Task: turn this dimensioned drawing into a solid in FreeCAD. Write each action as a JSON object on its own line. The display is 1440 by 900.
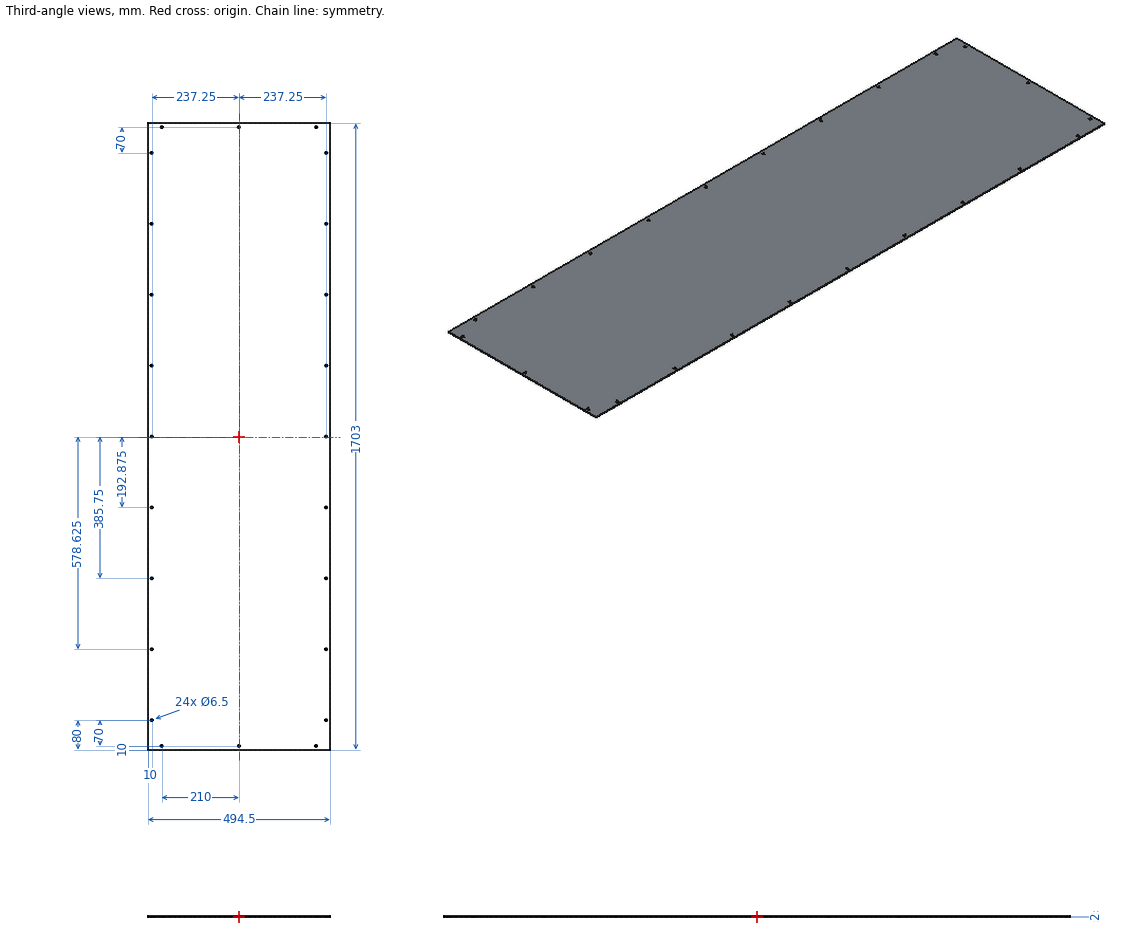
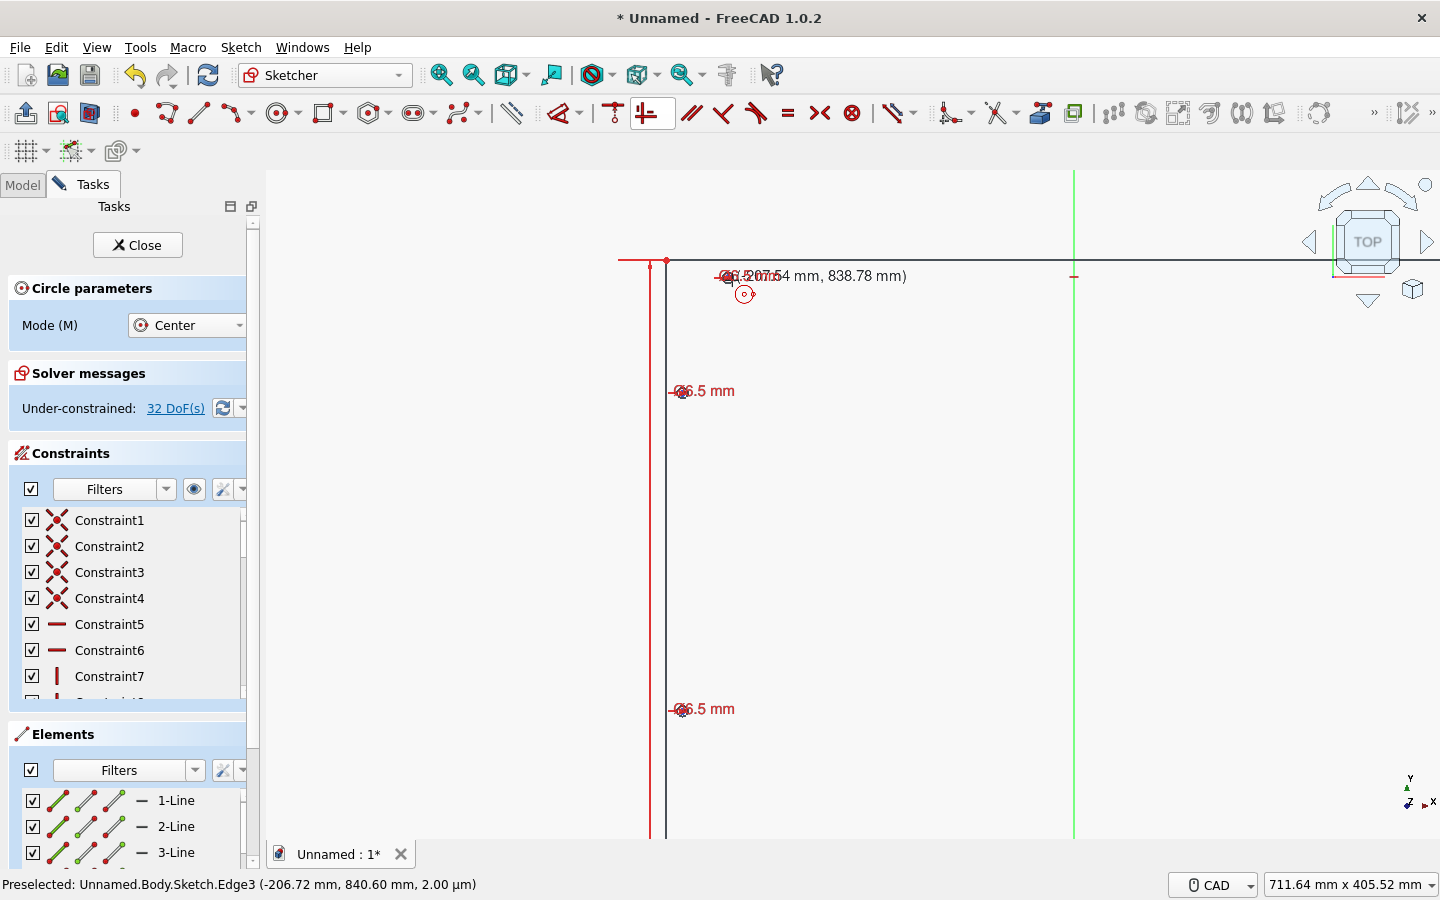
{"action": "scroll", "coordinate": [727, 275], "scroll_direction": "down", "scroll_amount": 9}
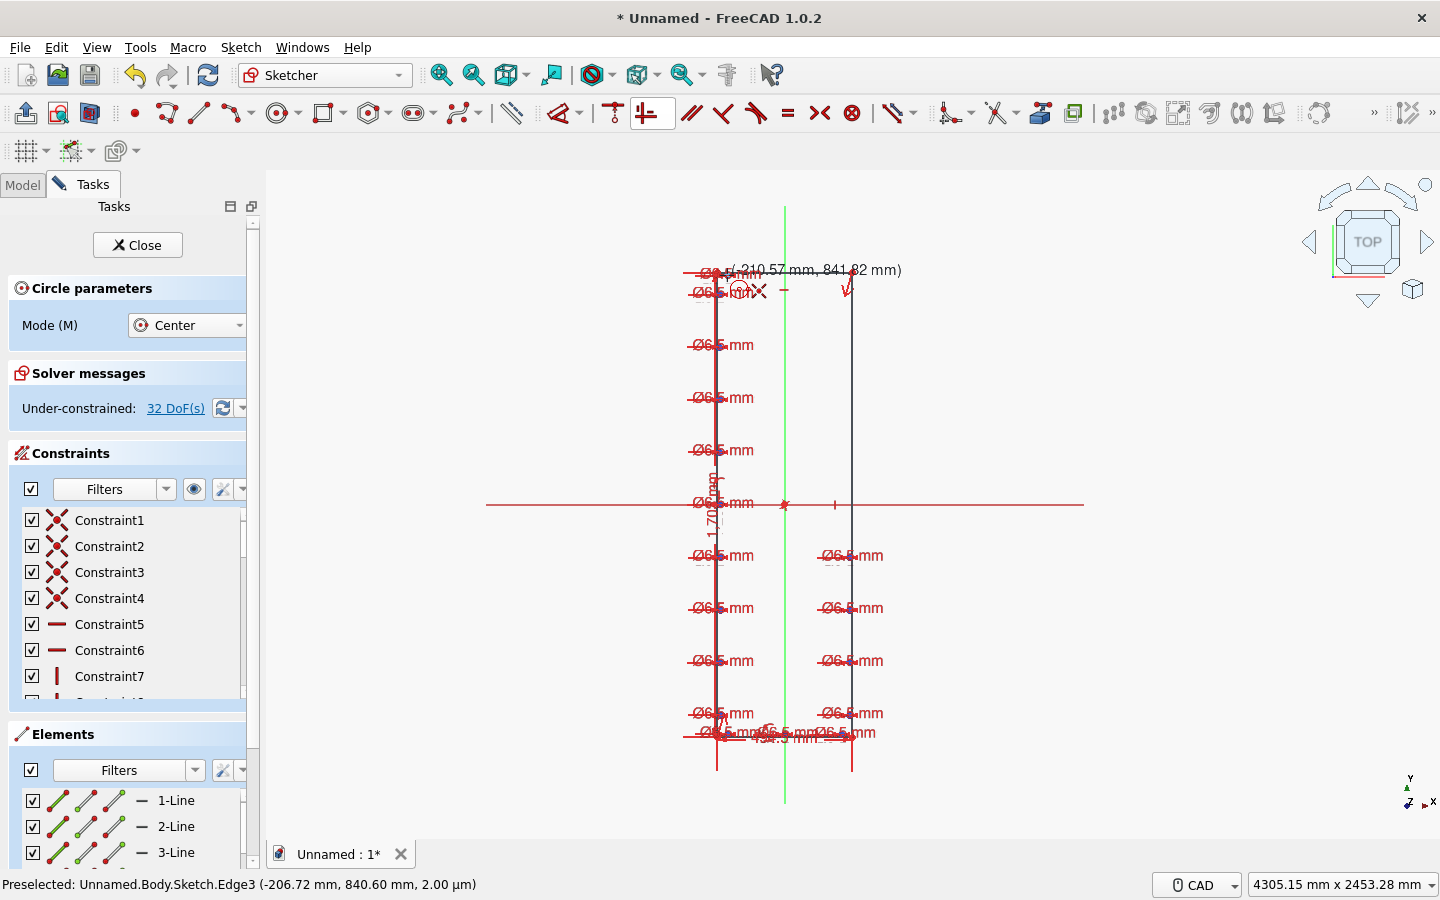
{"action": "scroll", "coordinate": [849, 505], "scroll_direction": "up", "scroll_amount": 17}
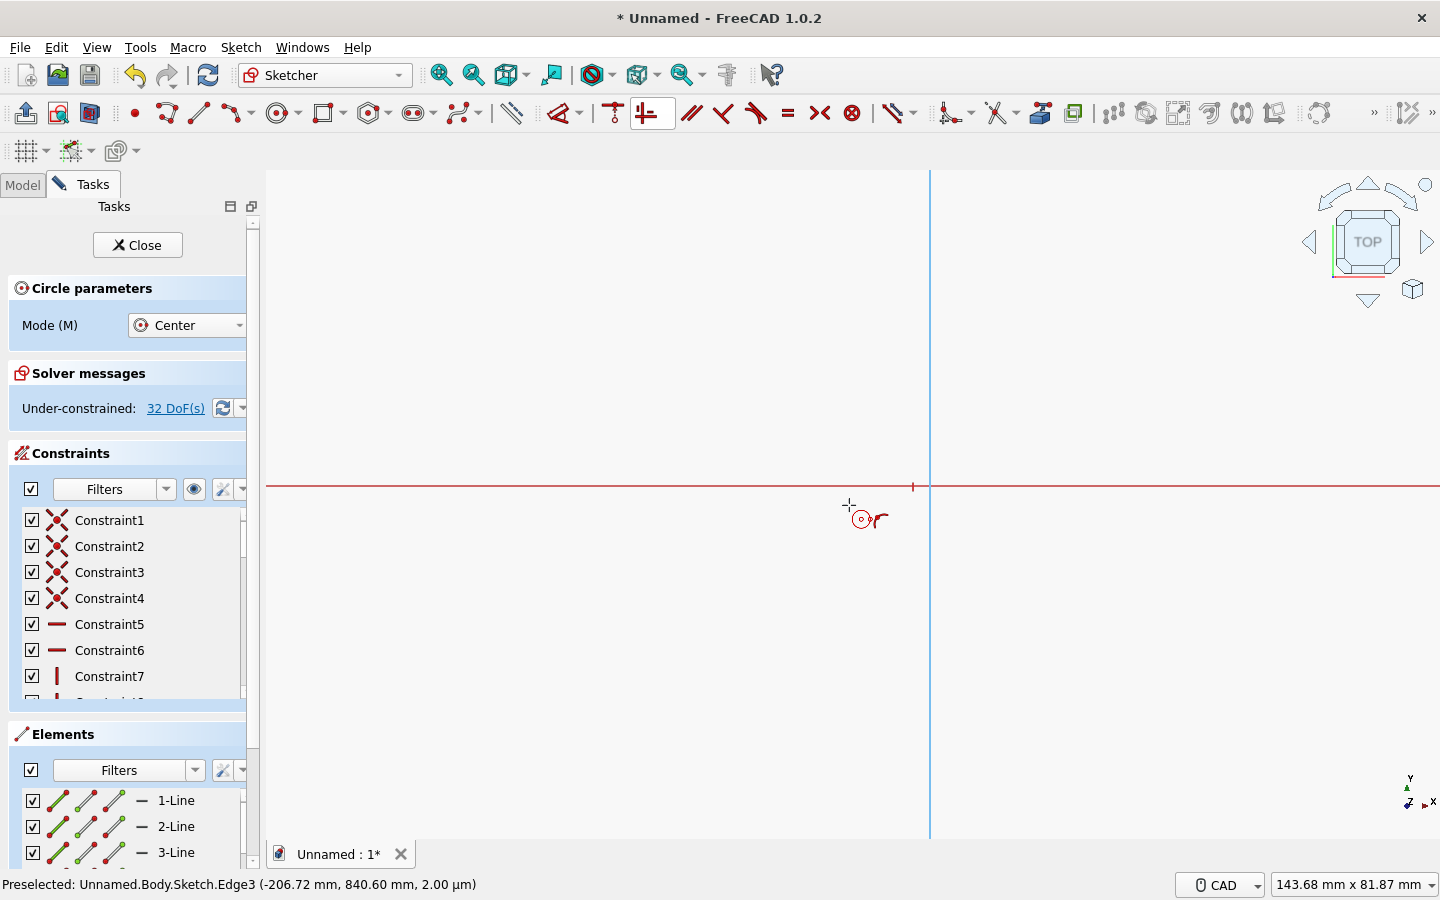
{"action": "scroll", "coordinate": [849, 505], "scroll_direction": "down", "scroll_amount": 17}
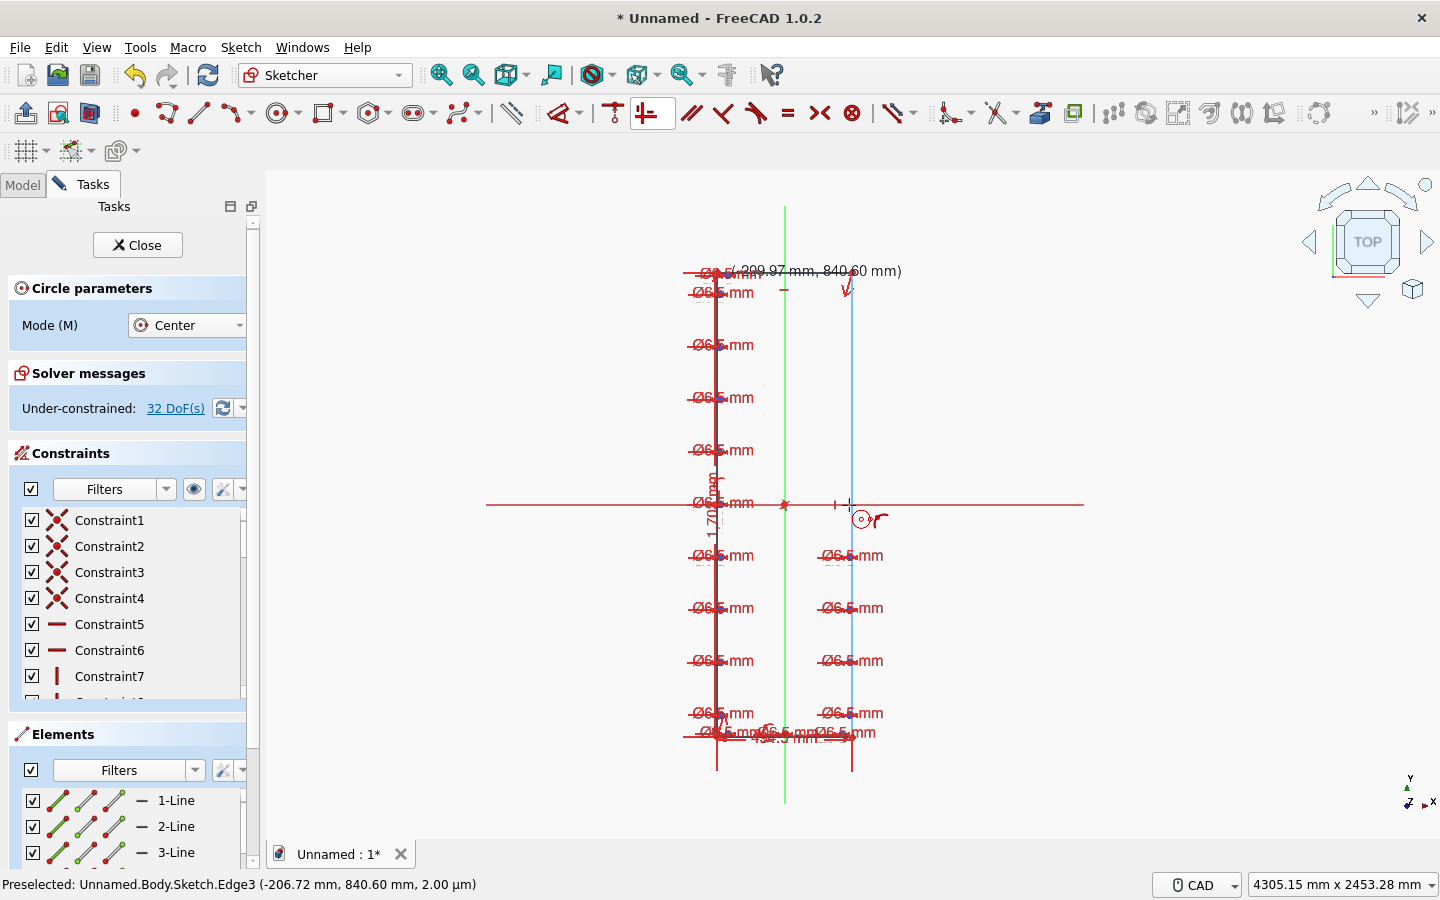
{"action": "scroll", "coordinate": [849, 505], "scroll_direction": "up", "scroll_amount": 9}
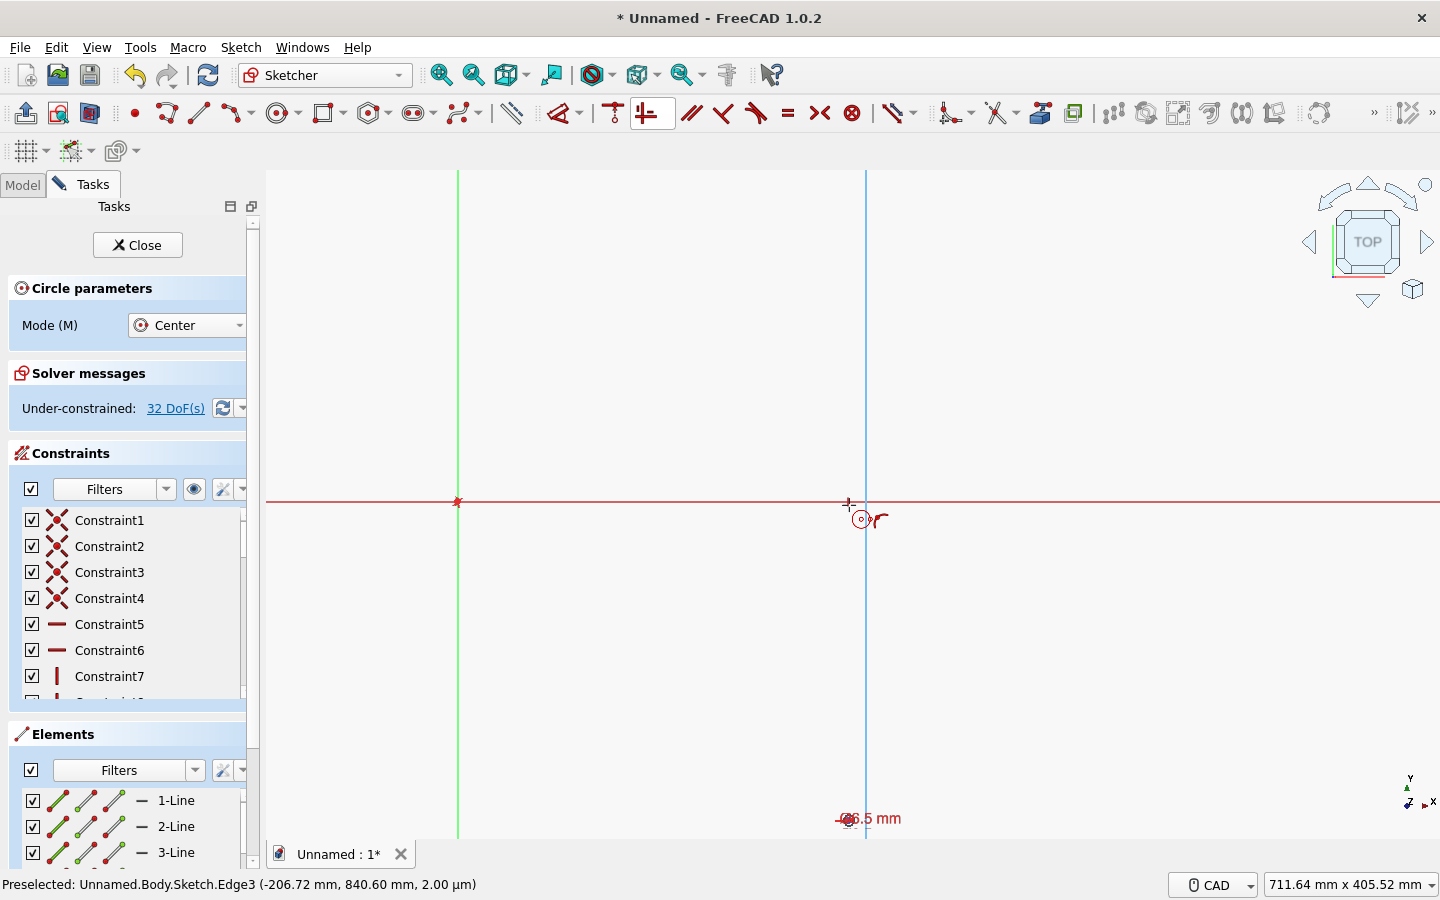
{"action": "left_click", "coordinate": [849, 502]}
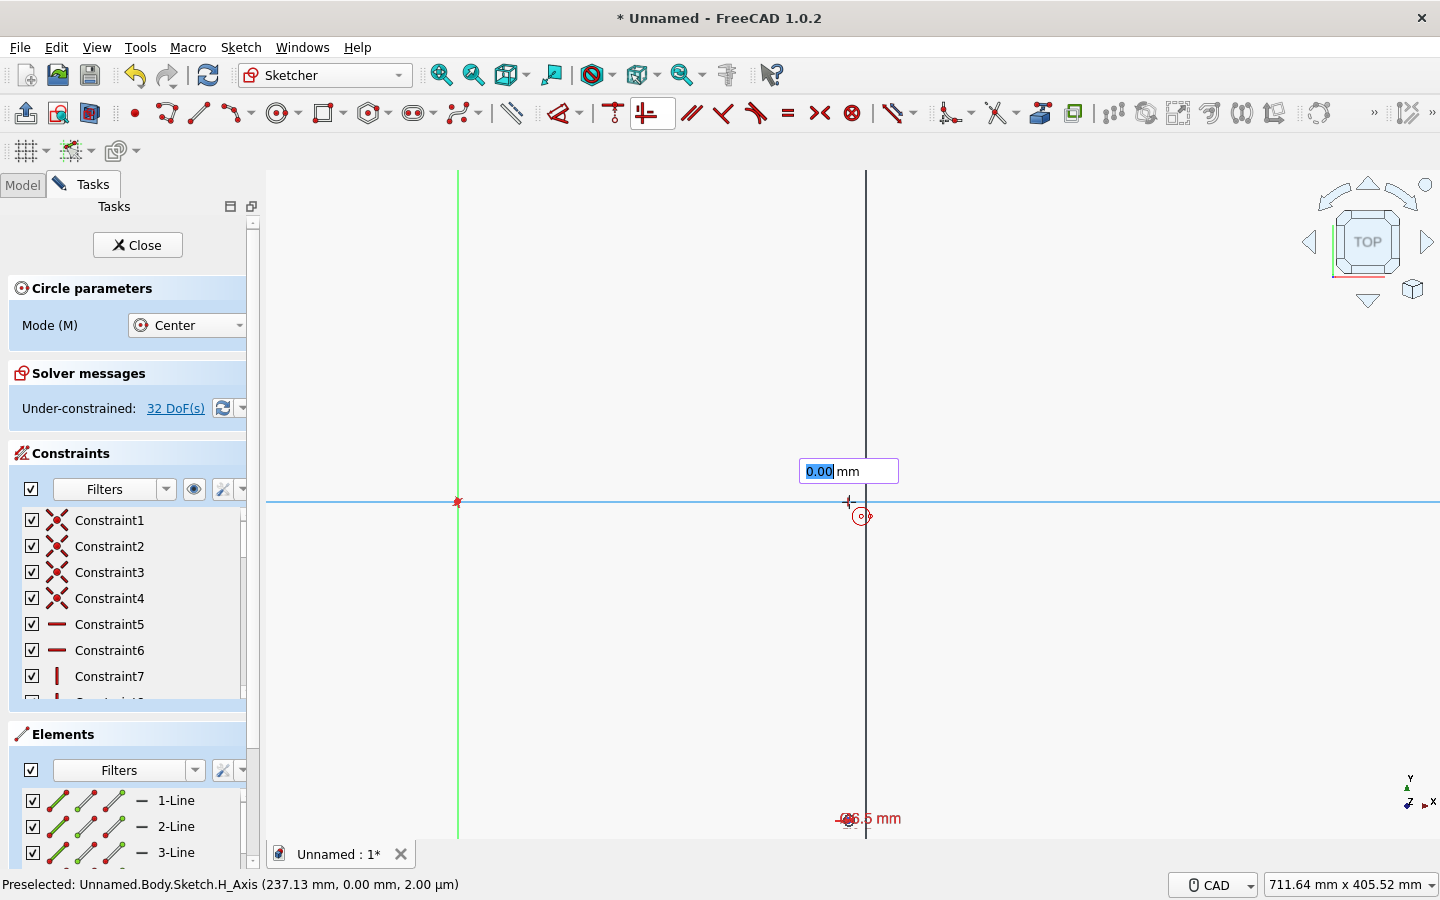
{"action": "scroll", "coordinate": [847, 507], "scroll_direction": "up", "scroll_amount": 6}
{"action": "mouse_move", "coordinate": [847, 505]}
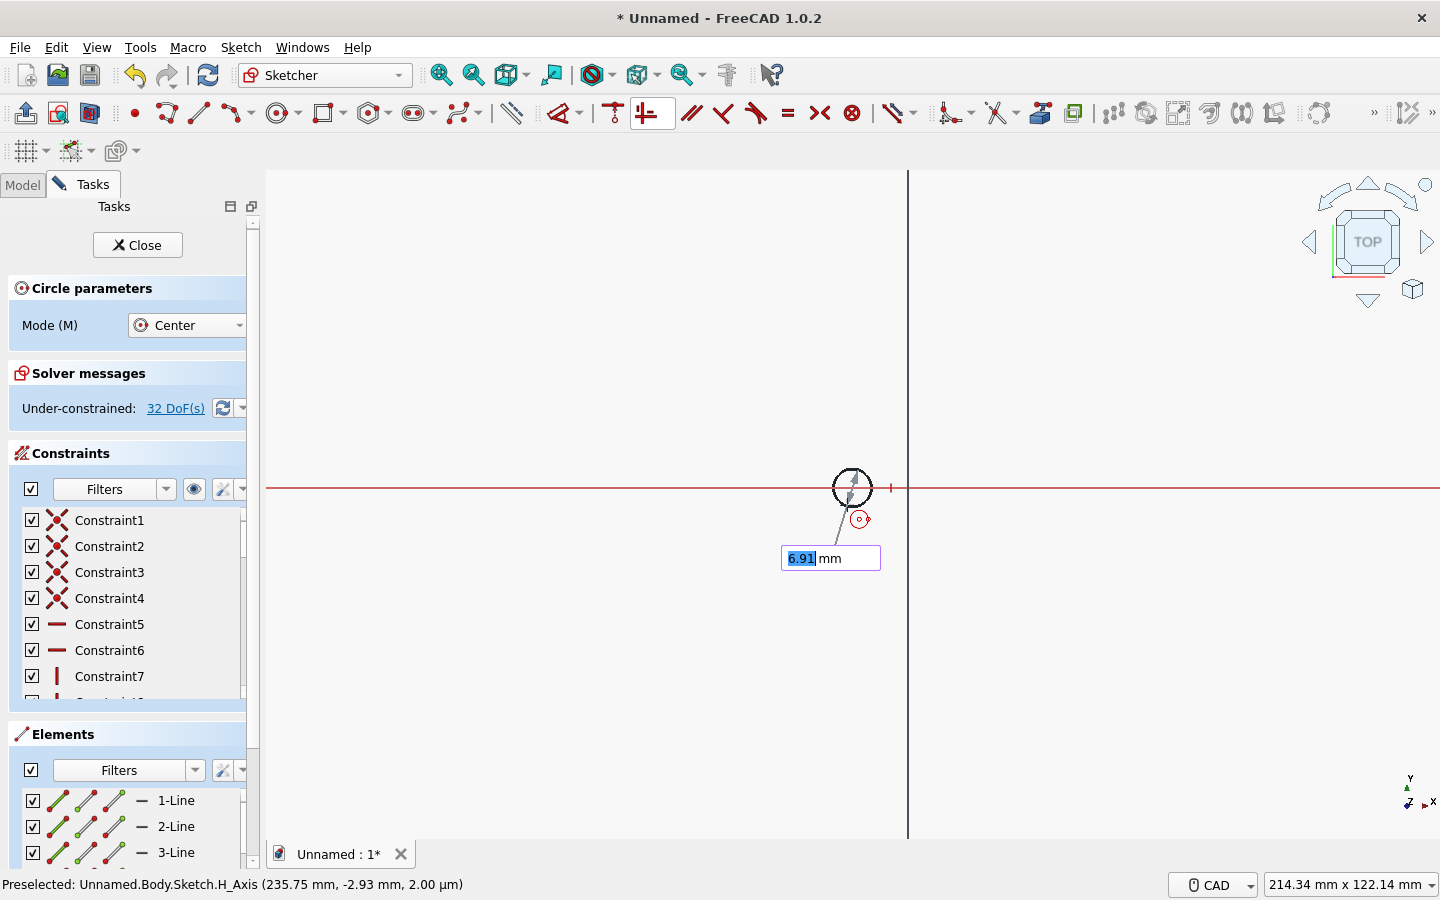
{"action": "type", "text": "6.5"}
{"action": "key", "text": "Return"}